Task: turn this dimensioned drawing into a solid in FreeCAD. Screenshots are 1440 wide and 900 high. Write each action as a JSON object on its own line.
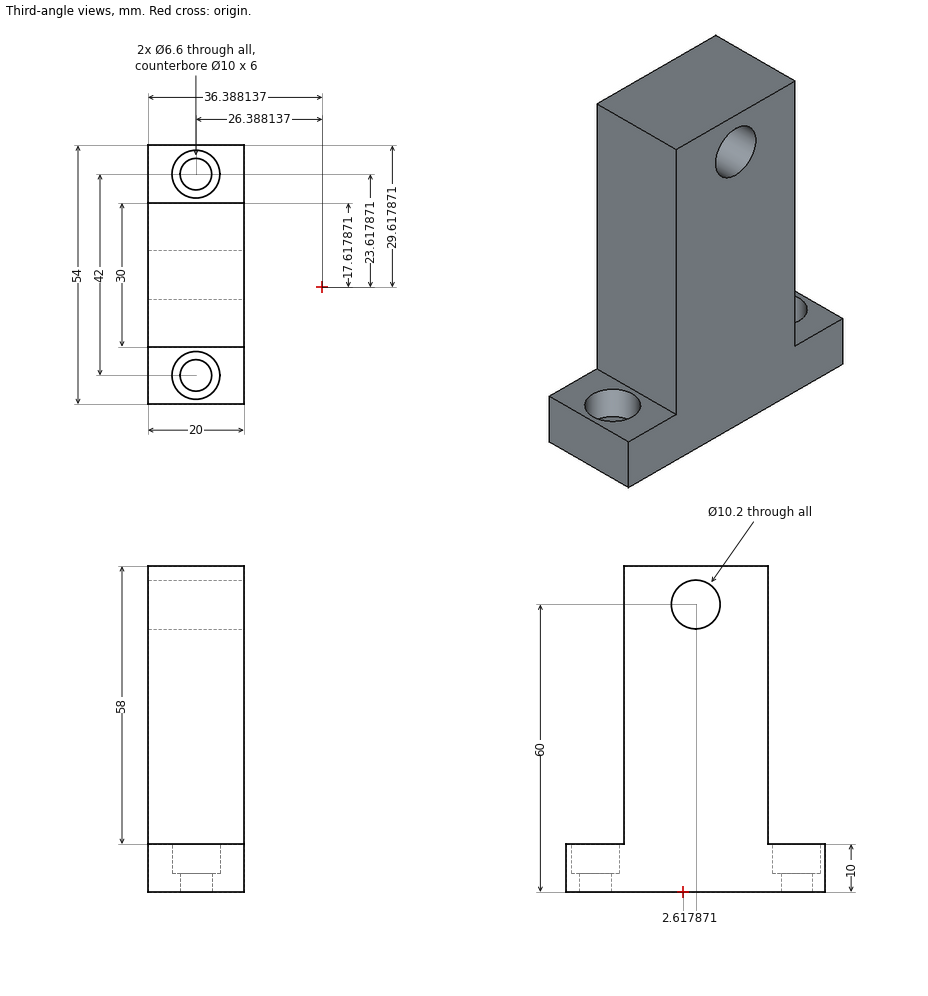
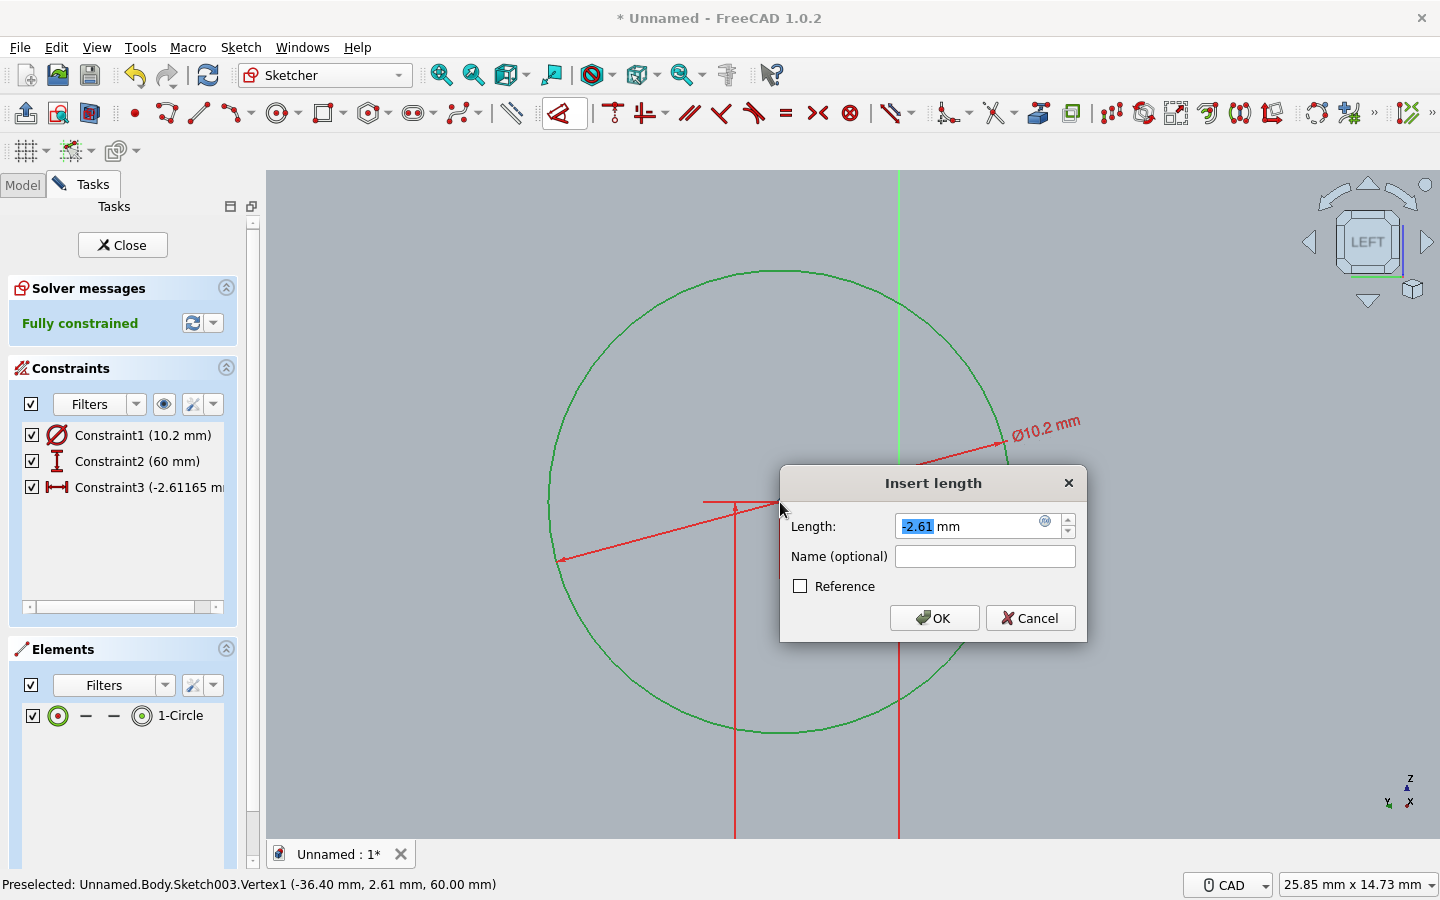
{"action": "type", "text": "-2.617871"}
{"action": "key", "text": "Return"}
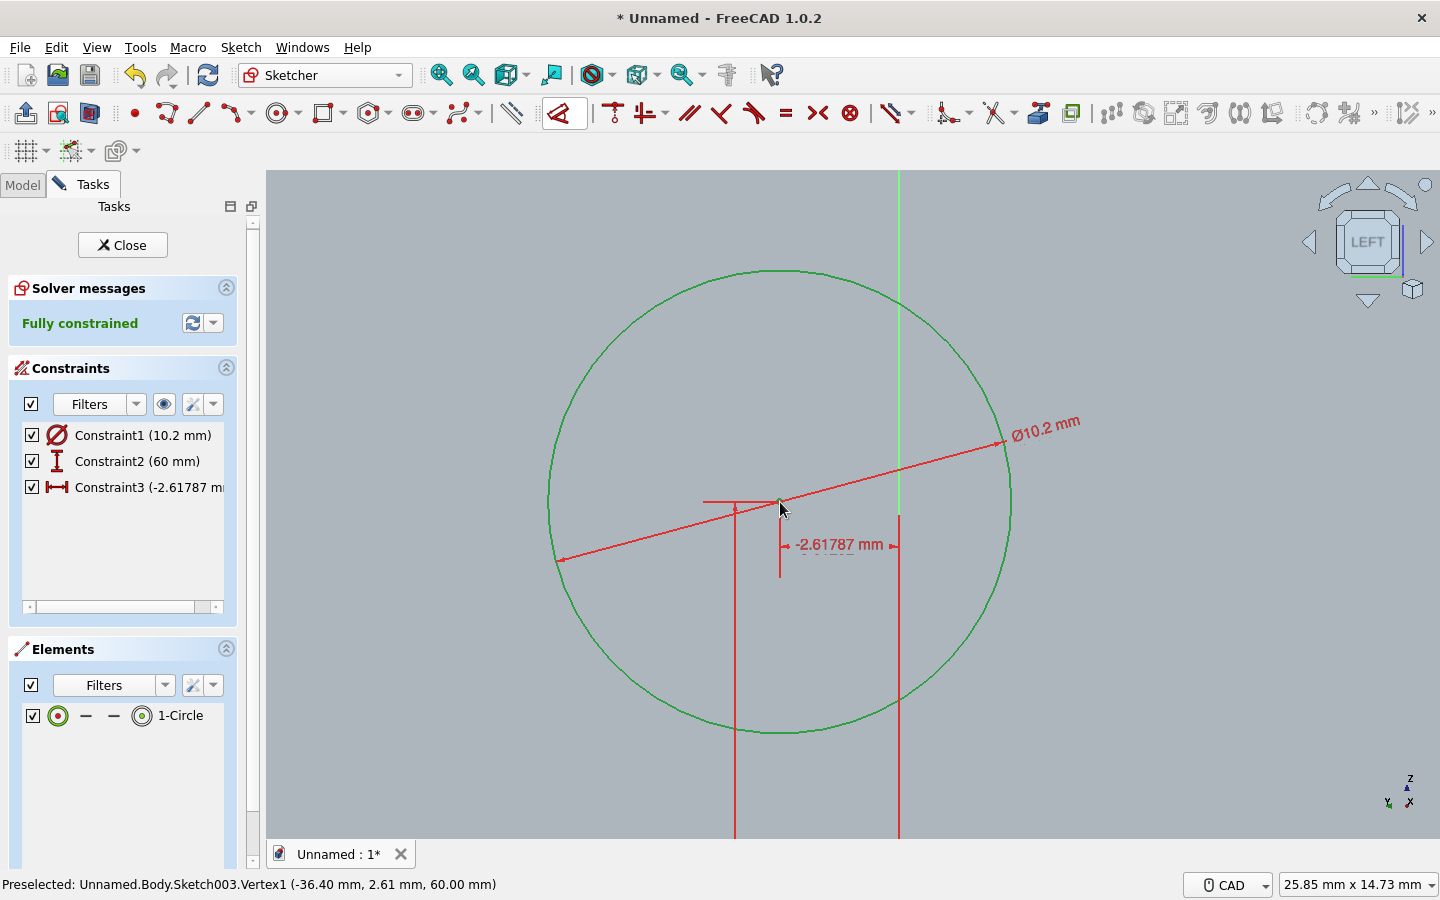
{"action": "left_click", "coordinate": [123, 245]}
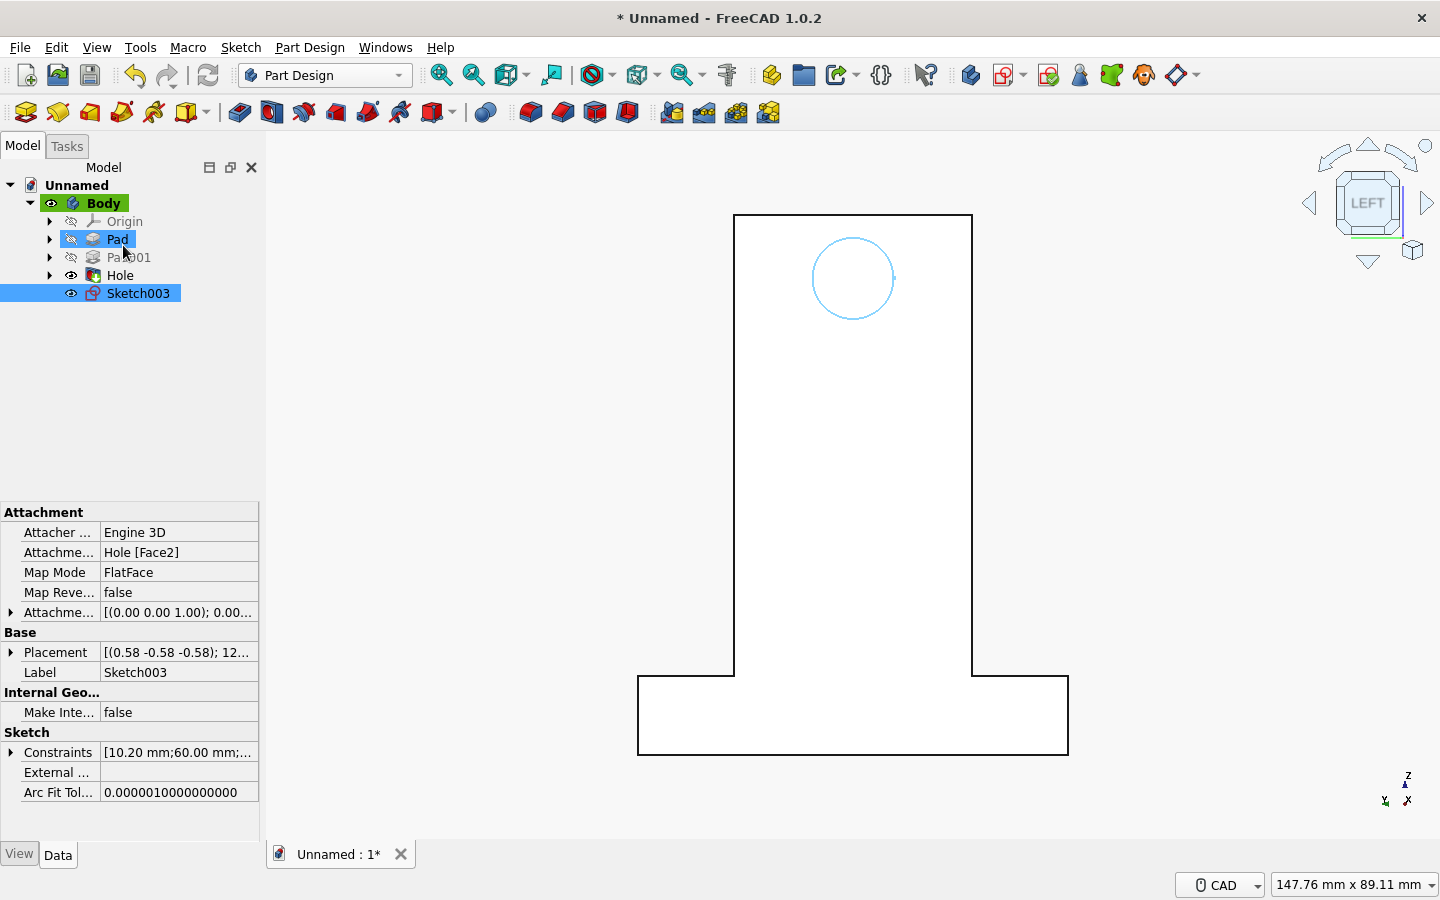
{"action": "left_click", "coordinate": [272, 112]}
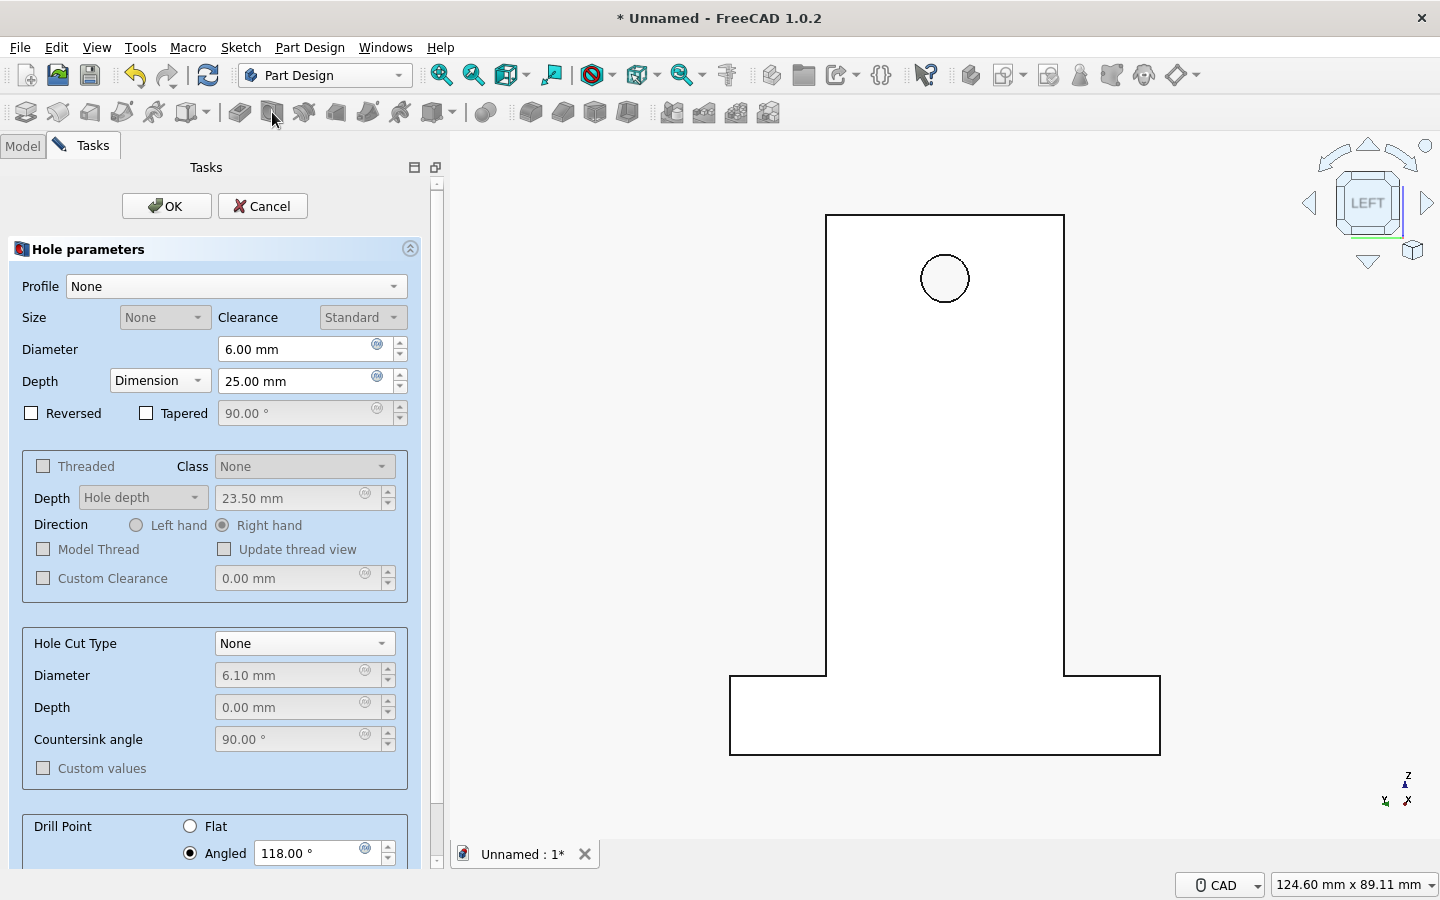
{"action": "triple_click", "coordinate": [305, 349]}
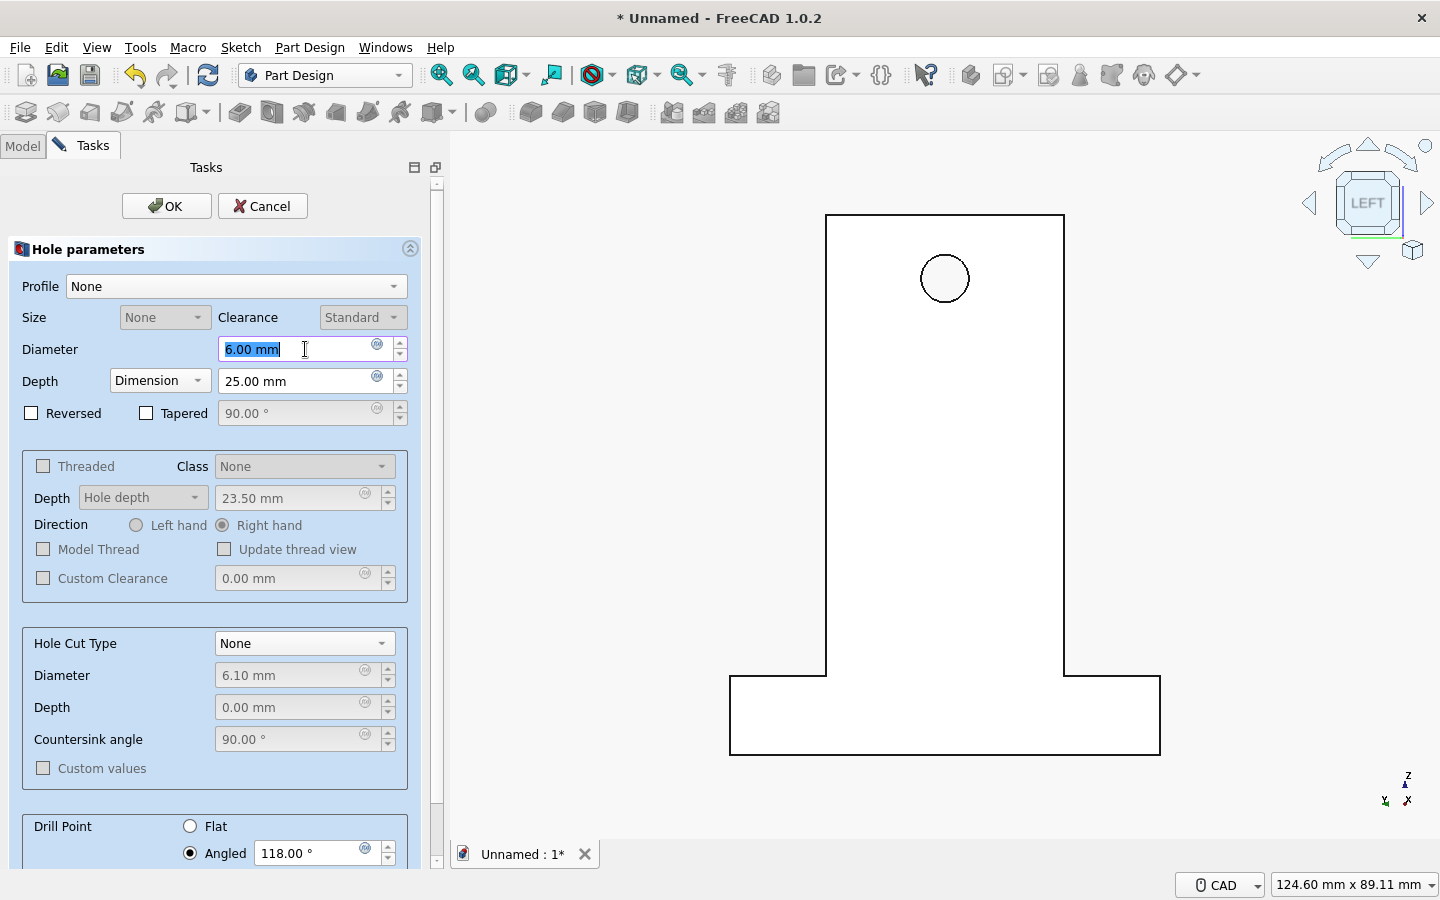
{"action": "type", "text": "10.2"}
{"action": "key", "text": "Tab"}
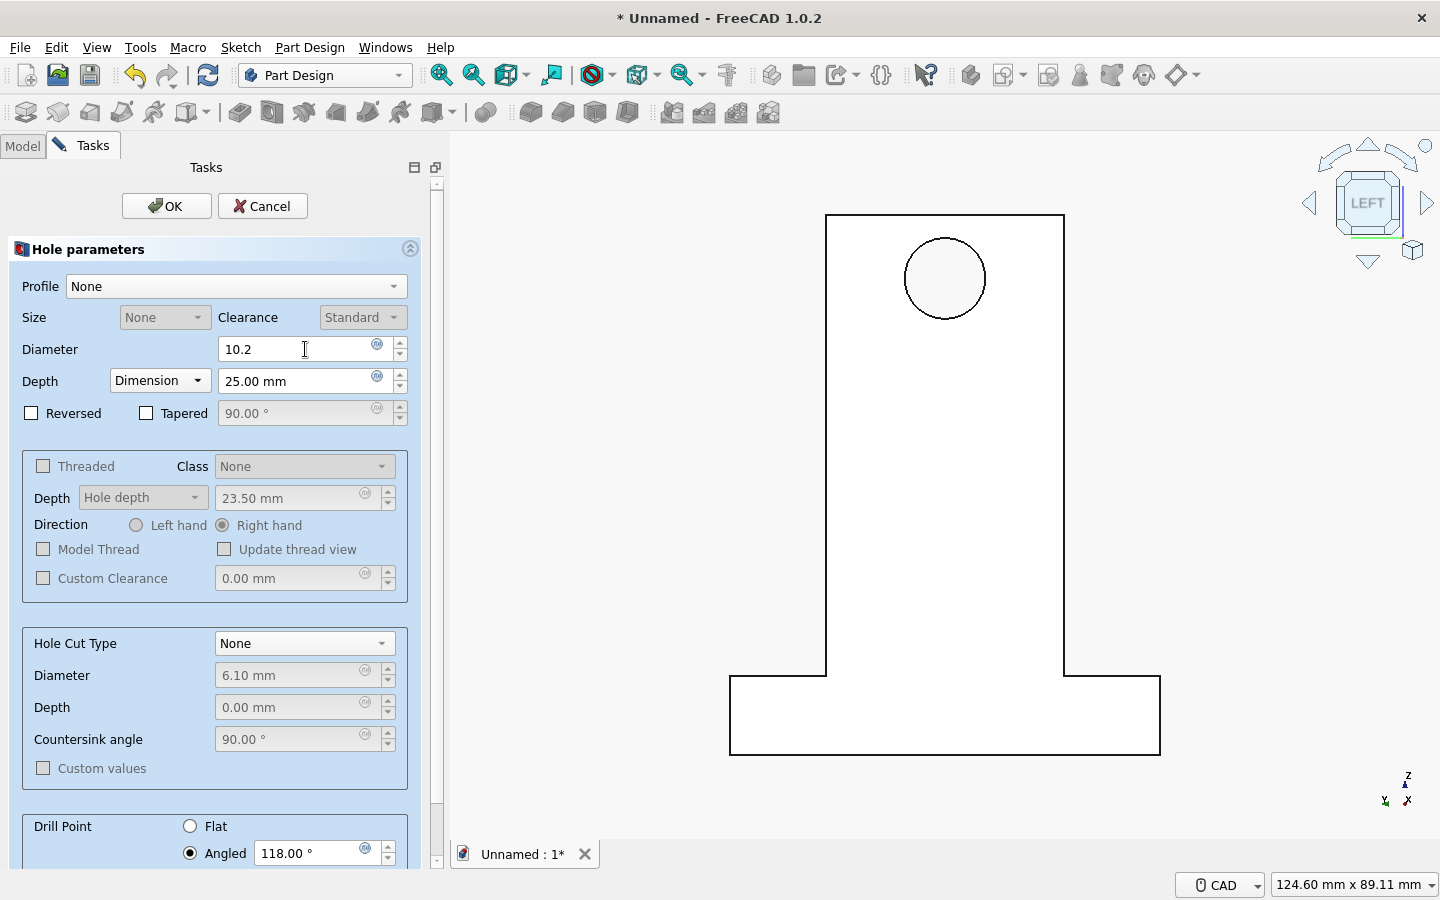
{"action": "left_click", "coordinate": [161, 380]}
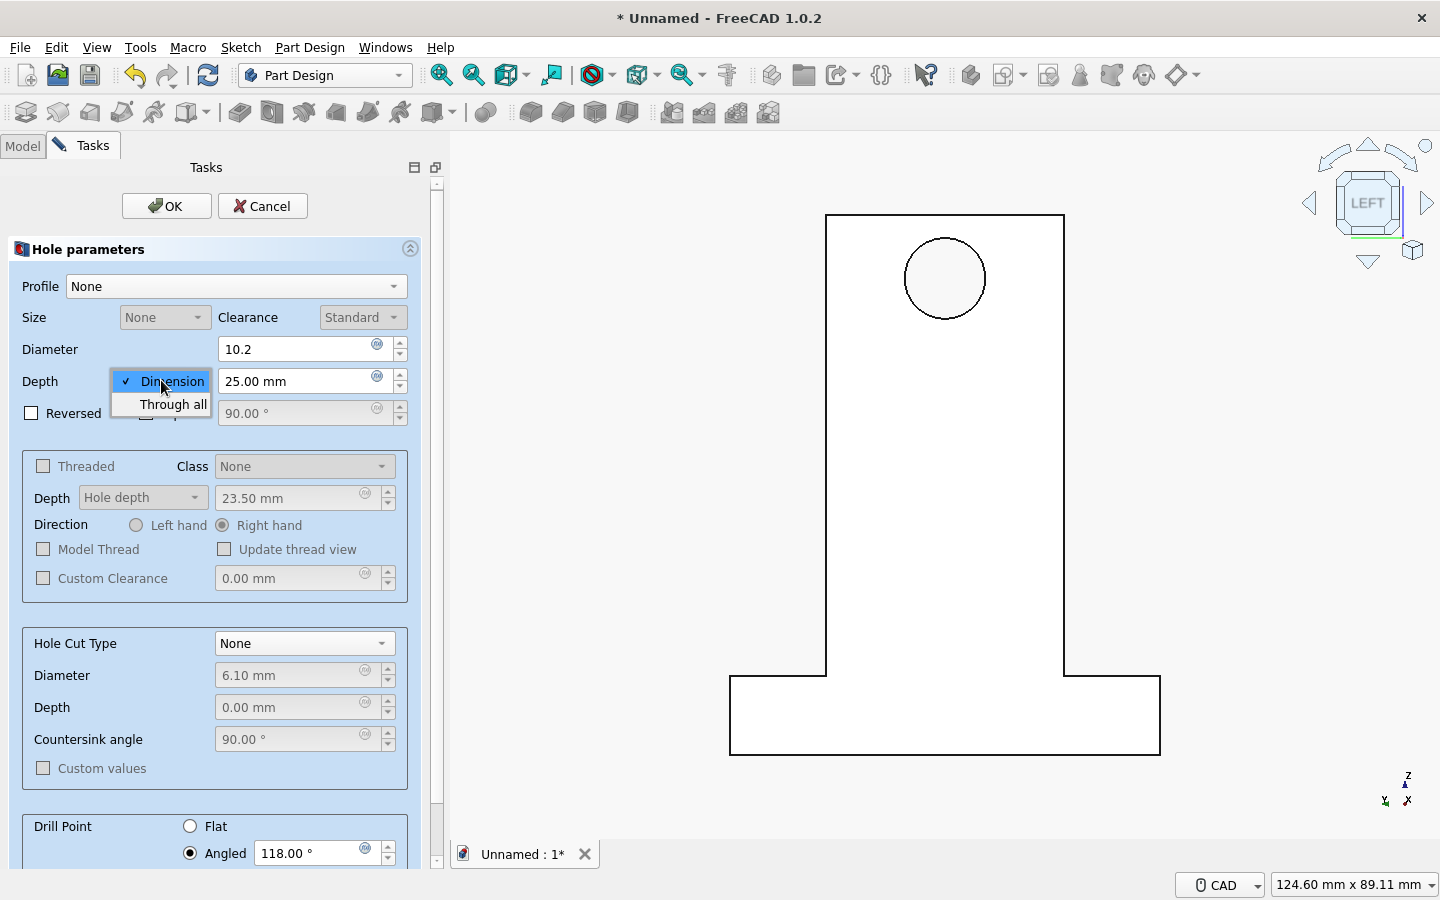
{"action": "left_click", "coordinate": [160, 404]}